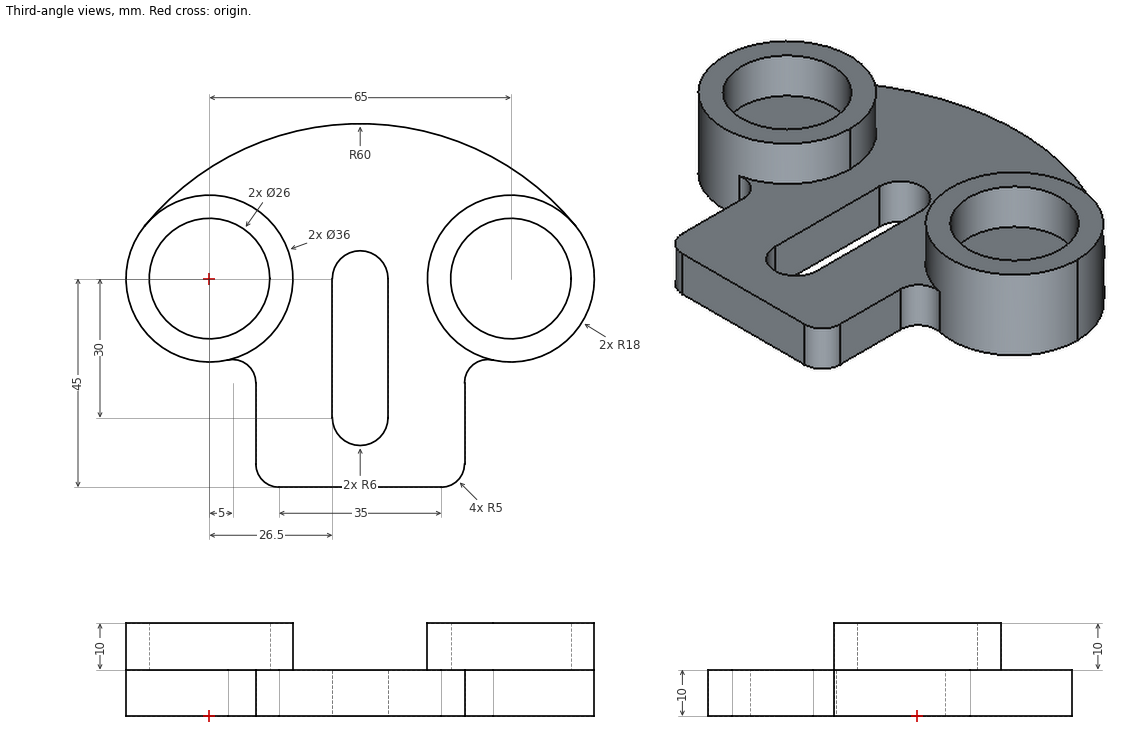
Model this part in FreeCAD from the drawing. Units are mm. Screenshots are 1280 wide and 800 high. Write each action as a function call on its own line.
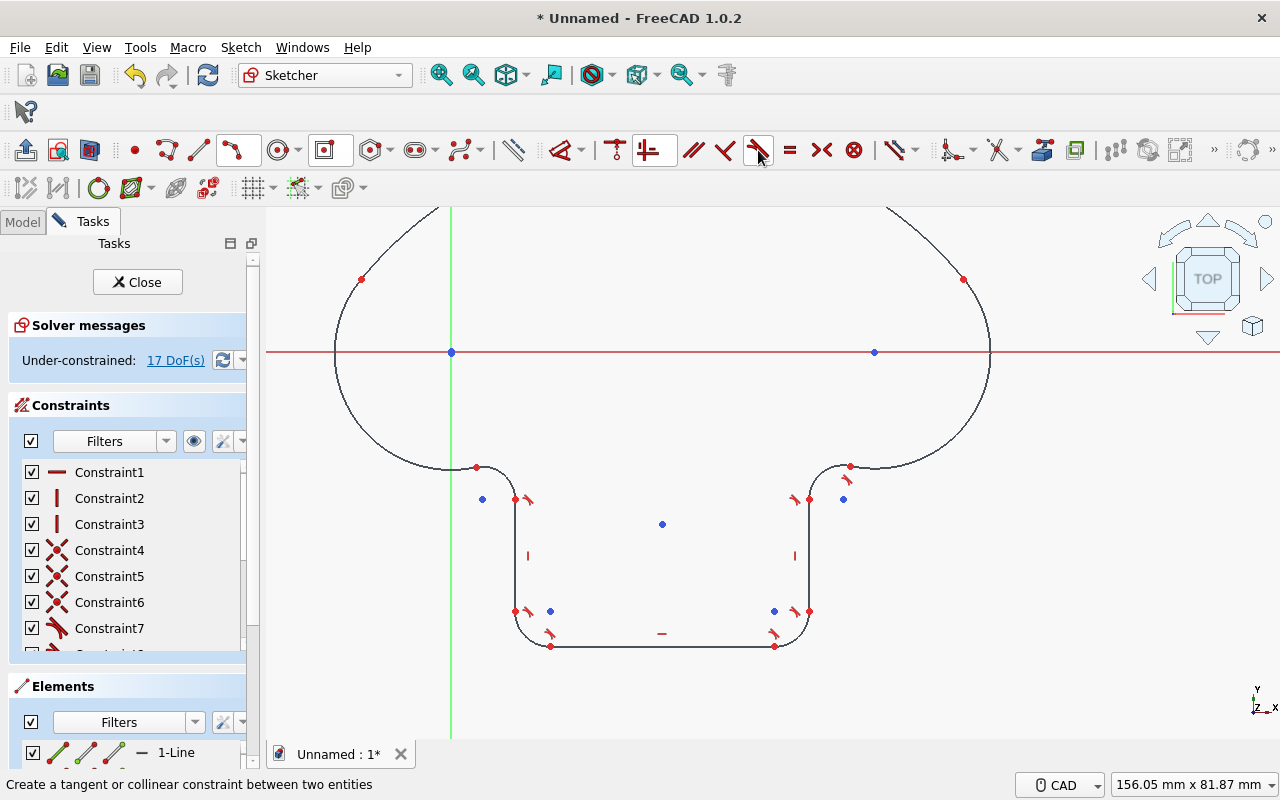
click(933, 453)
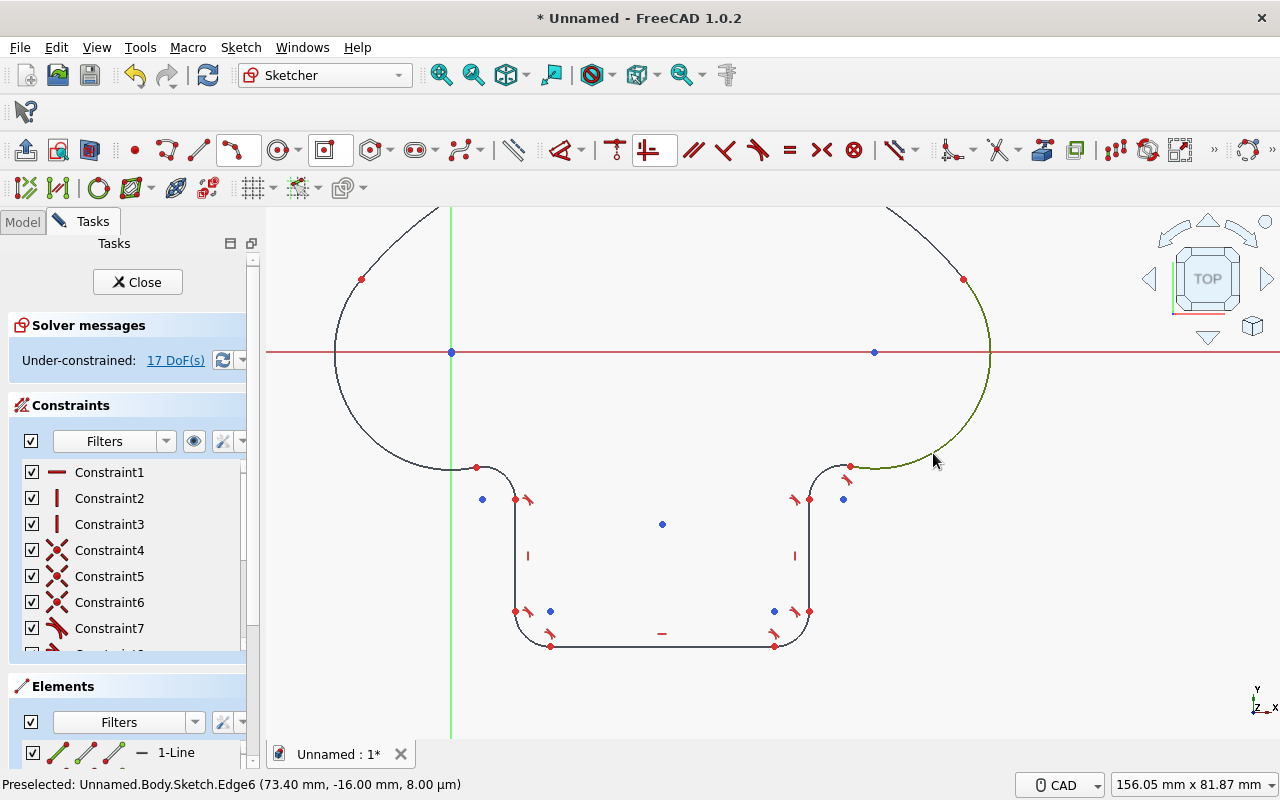
scroll(790, 643, down, 2)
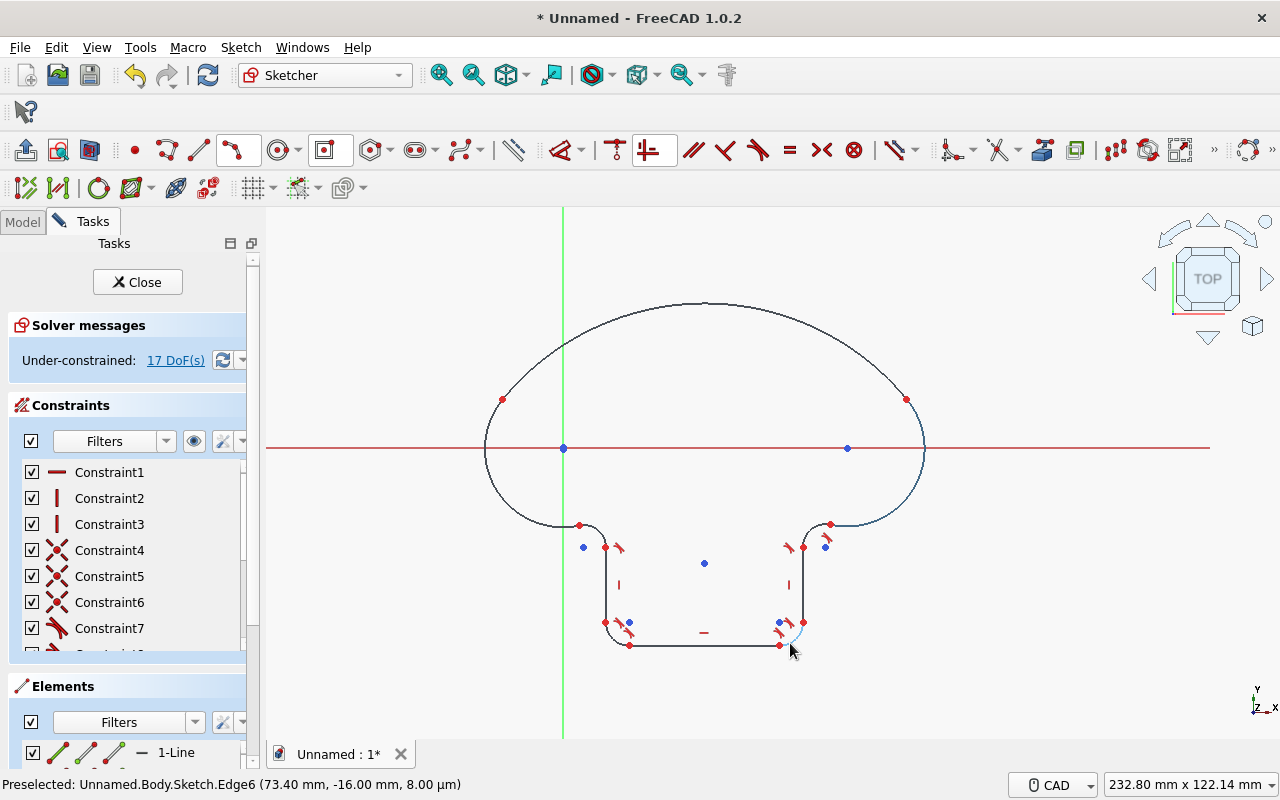
click(795, 320)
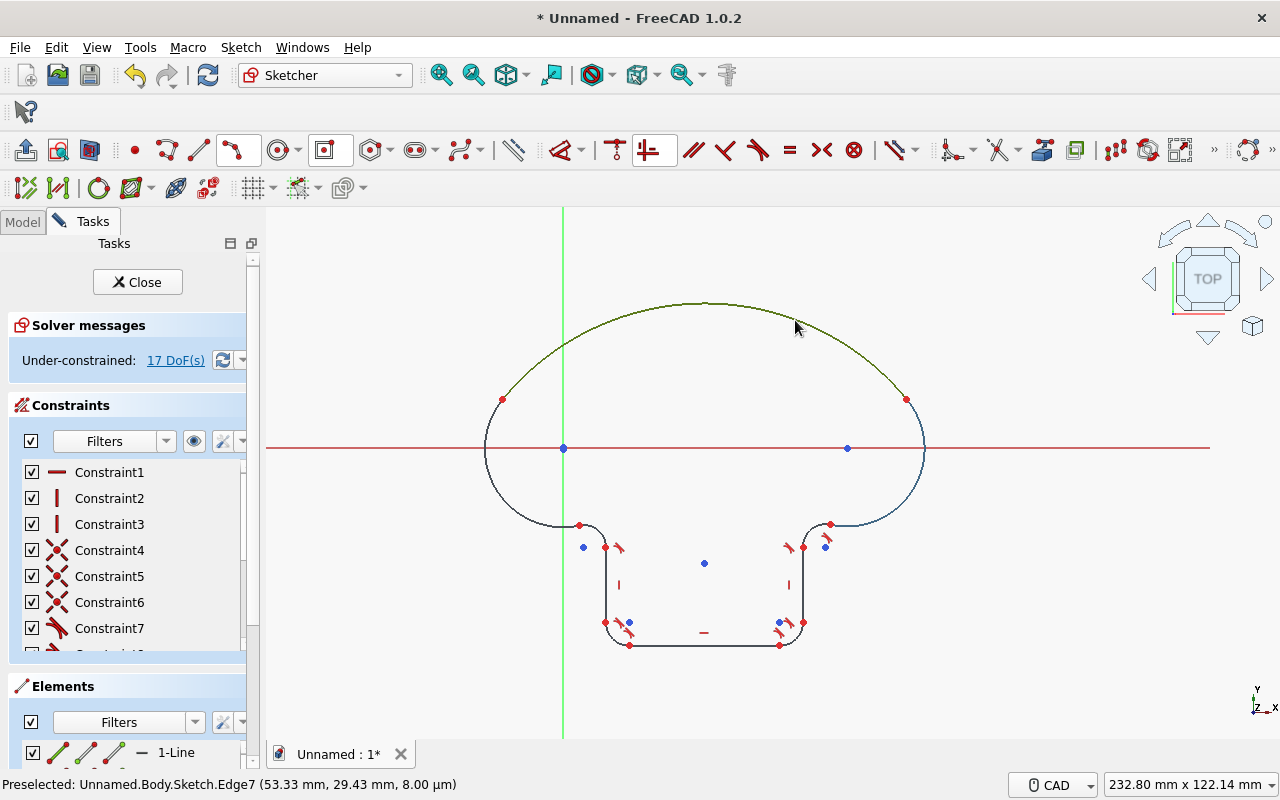
click(758, 150)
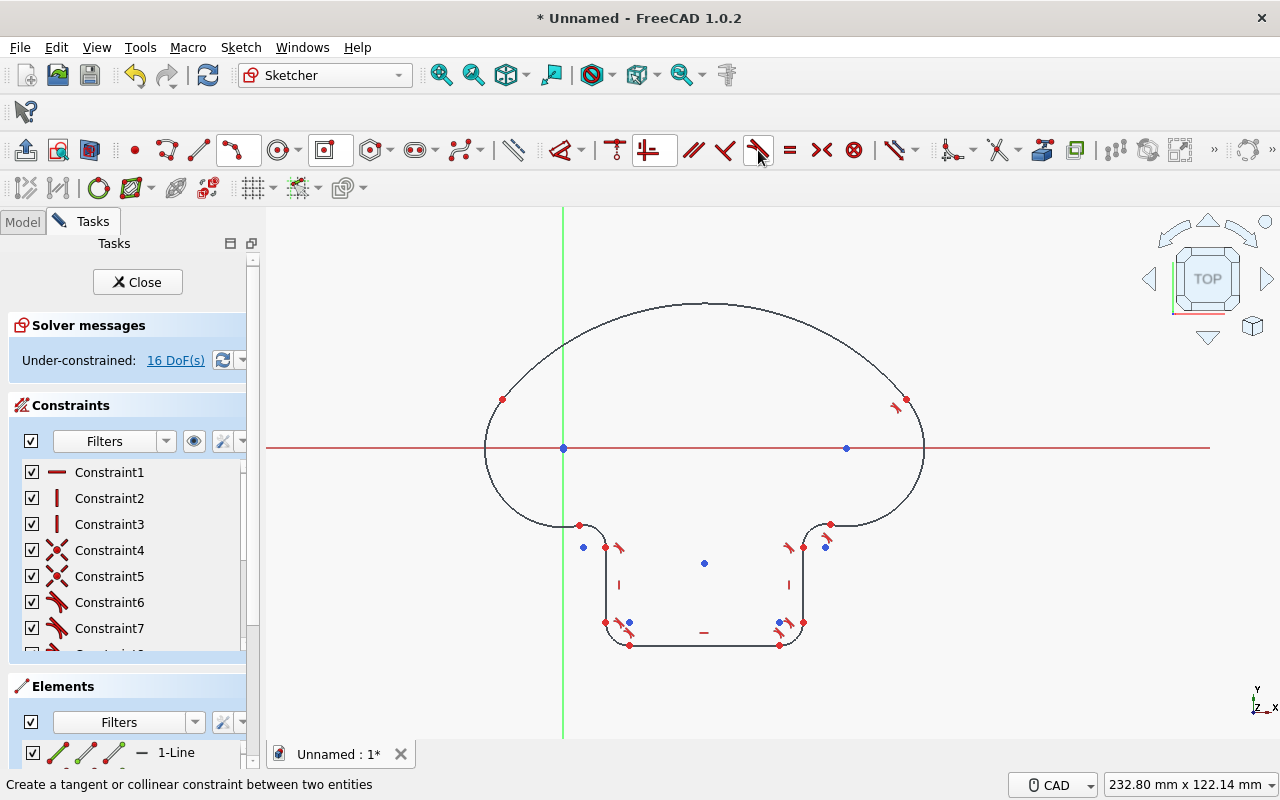
click(795, 320)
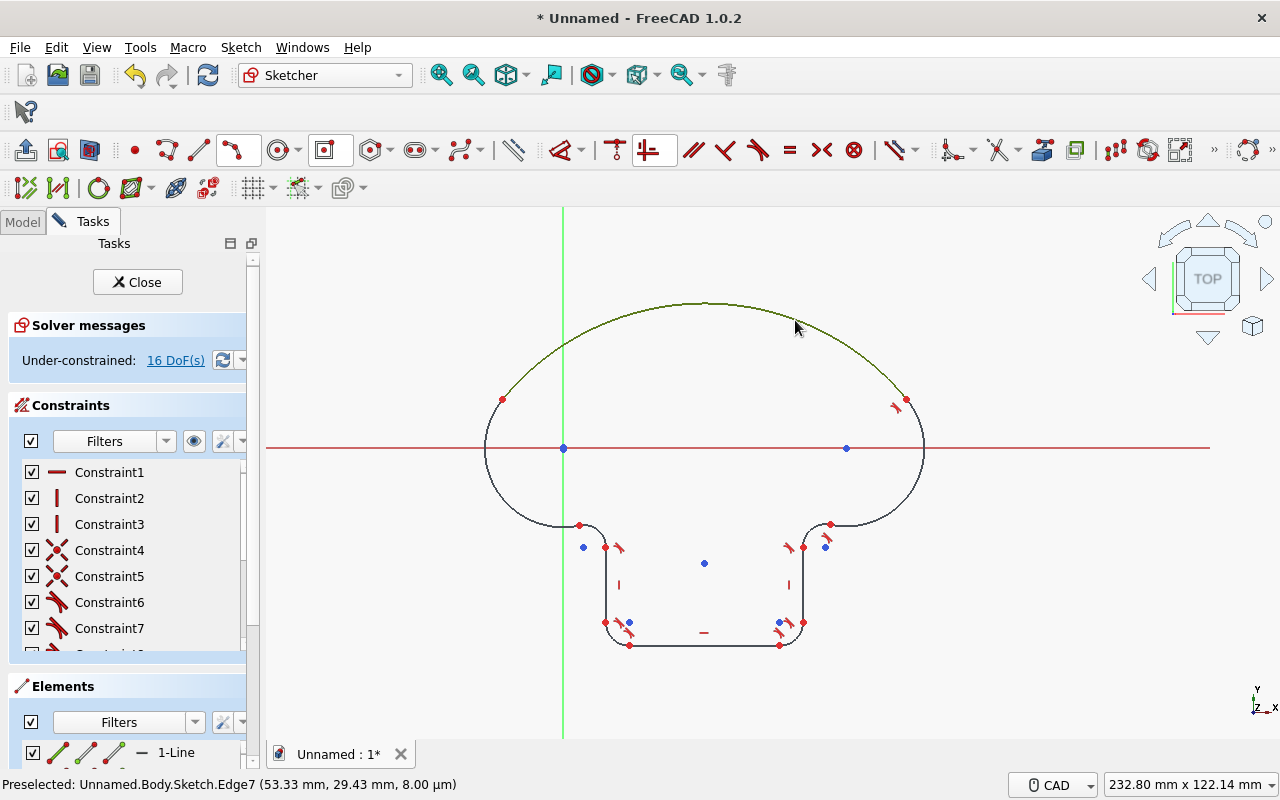
click(524, 517)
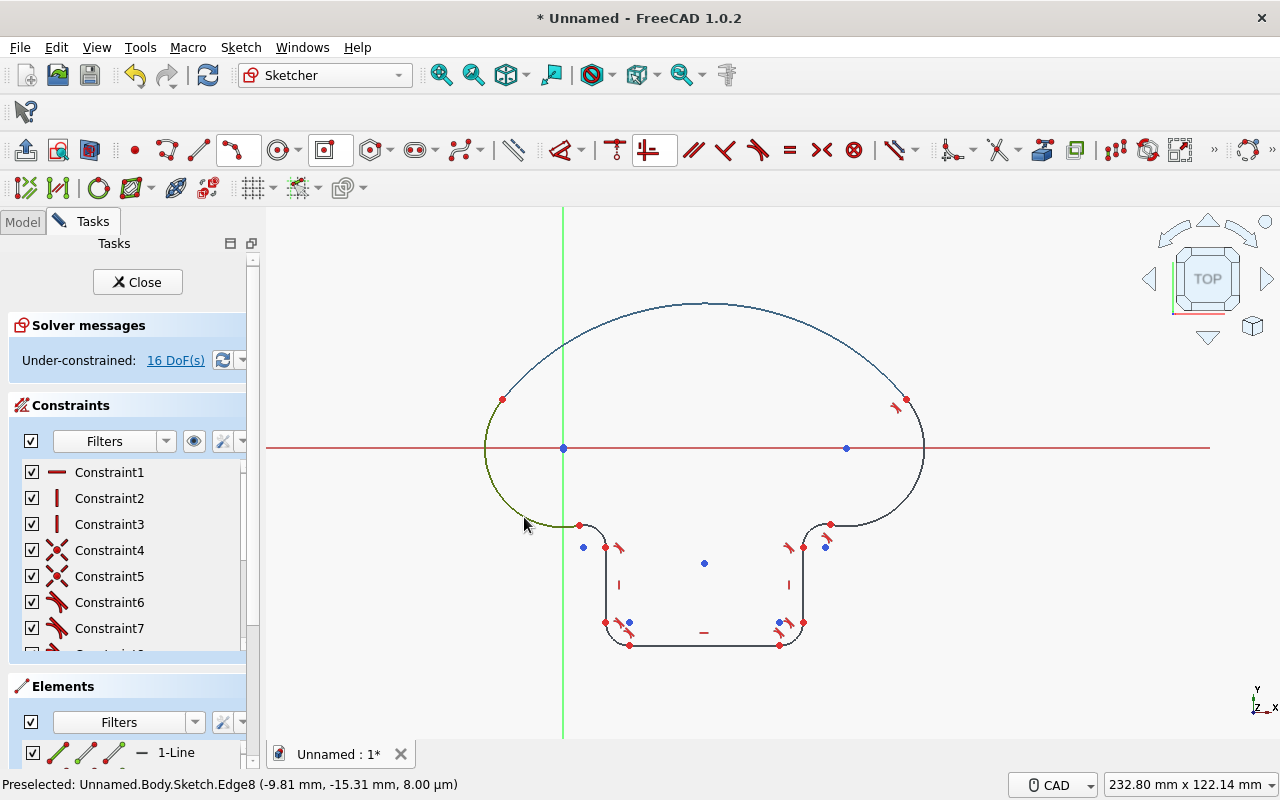
click(758, 150)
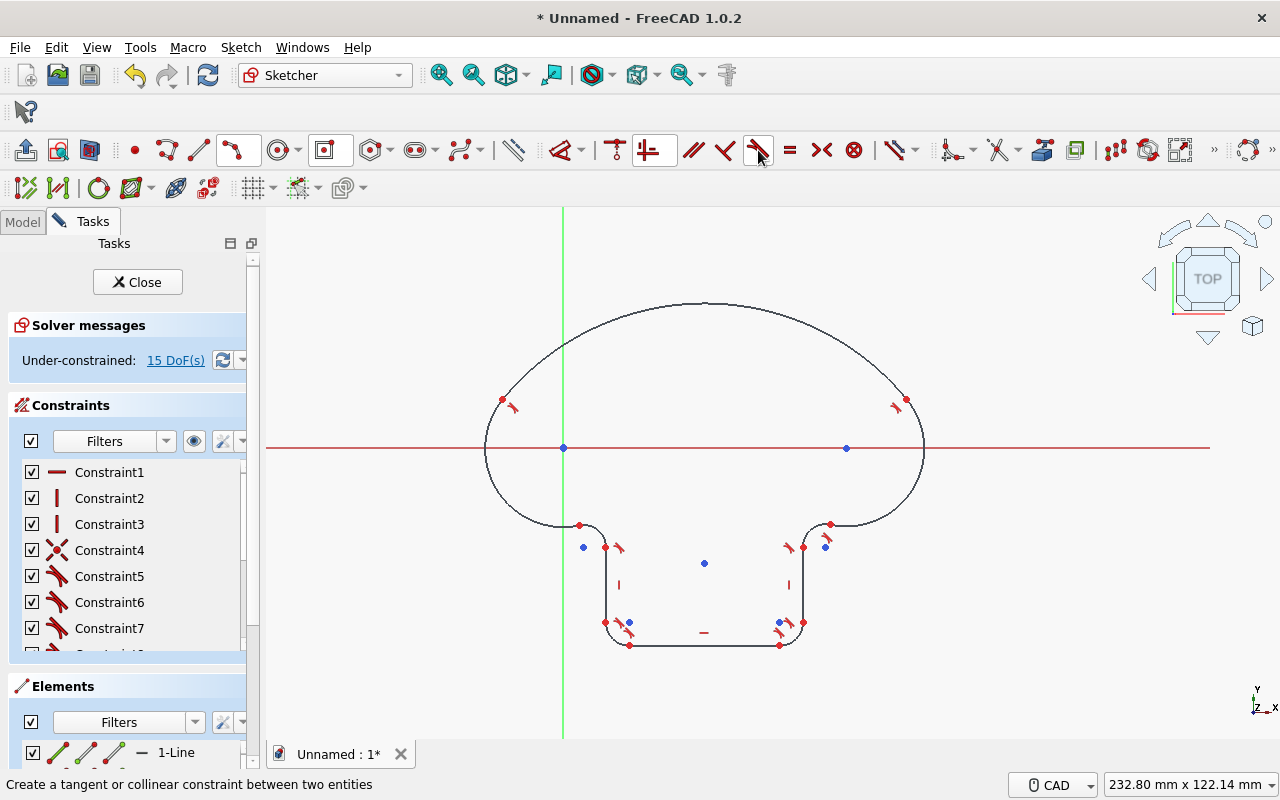
click(524, 516)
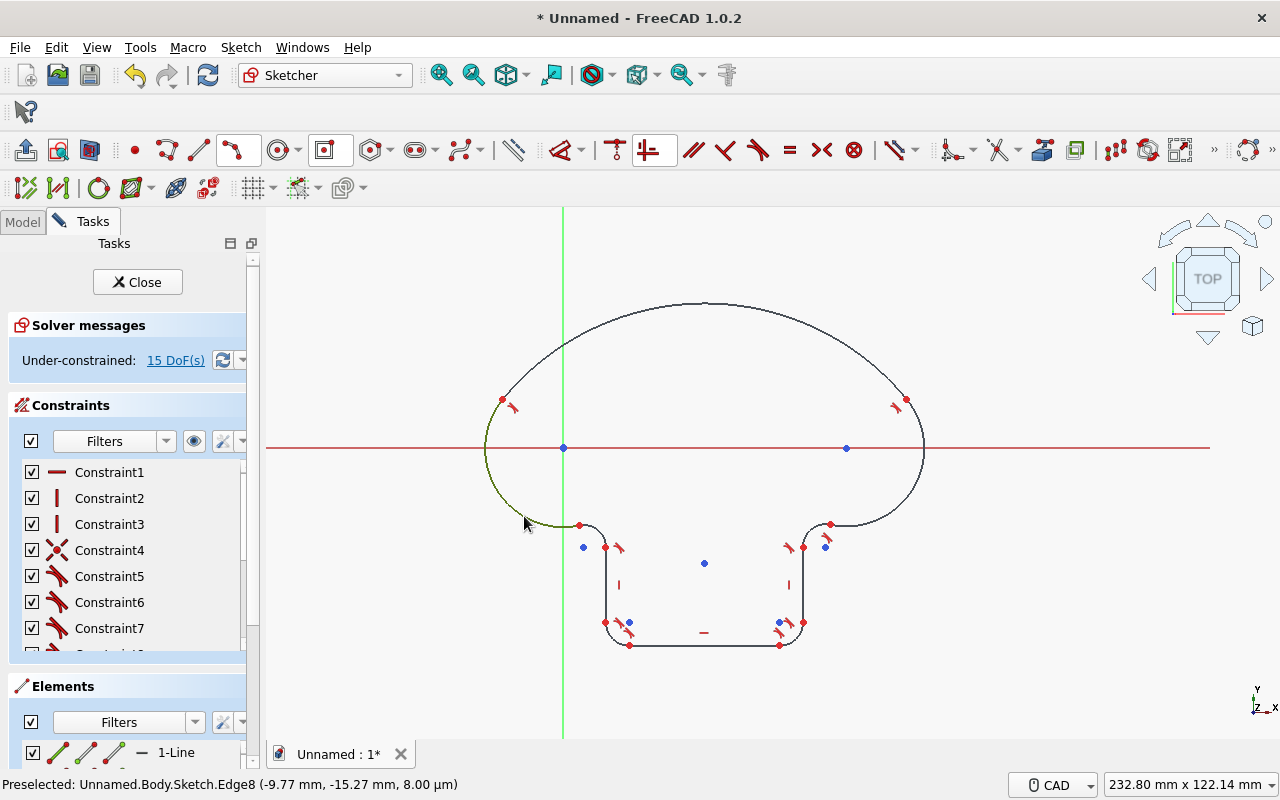
click(603, 536)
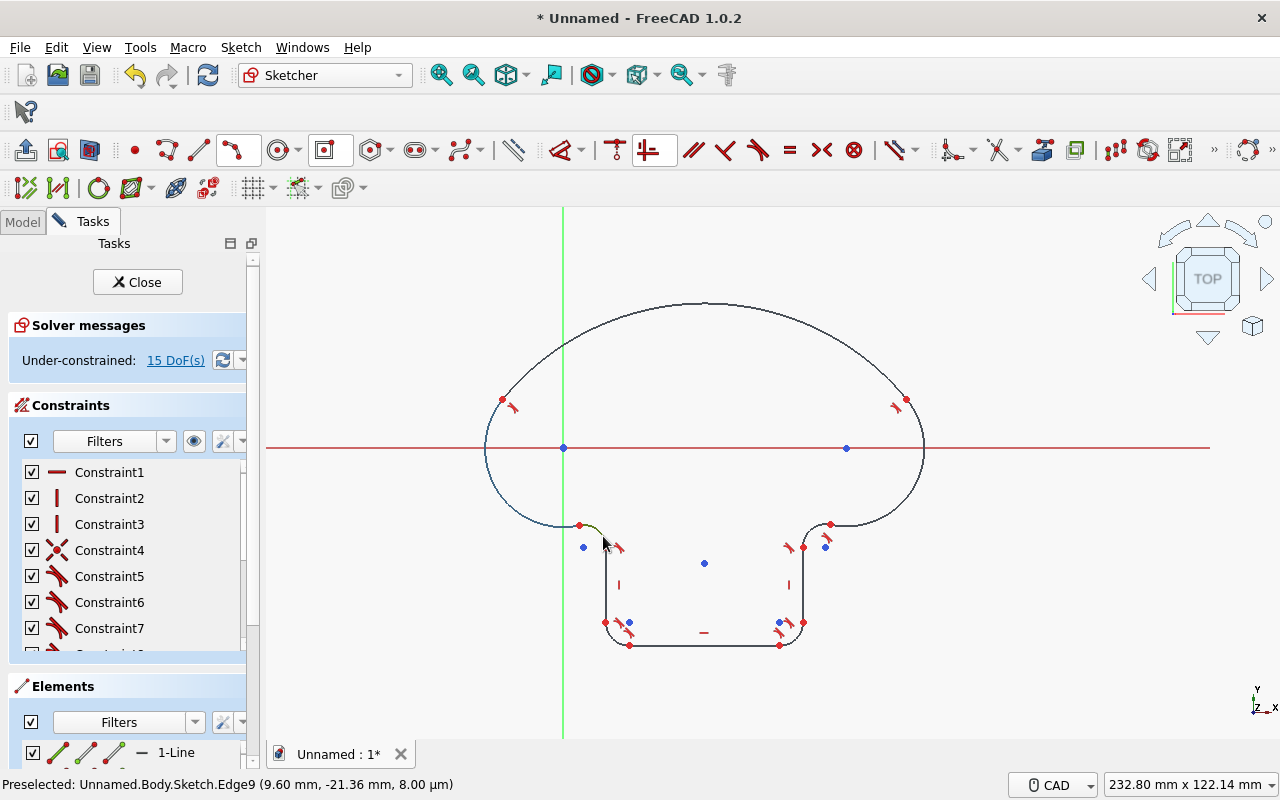
click(758, 150)